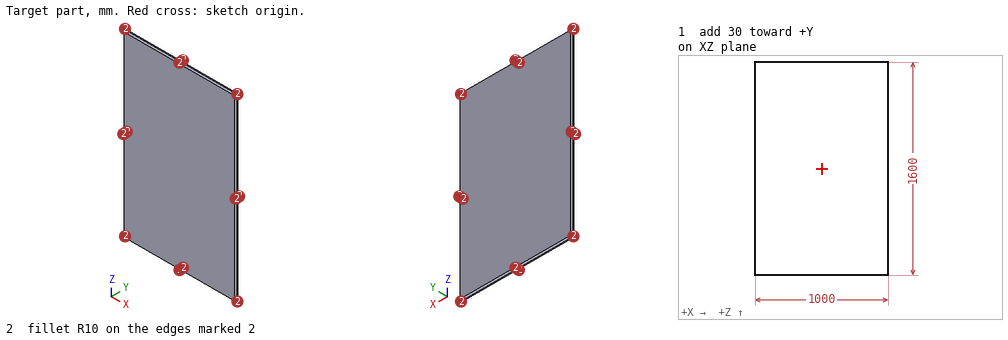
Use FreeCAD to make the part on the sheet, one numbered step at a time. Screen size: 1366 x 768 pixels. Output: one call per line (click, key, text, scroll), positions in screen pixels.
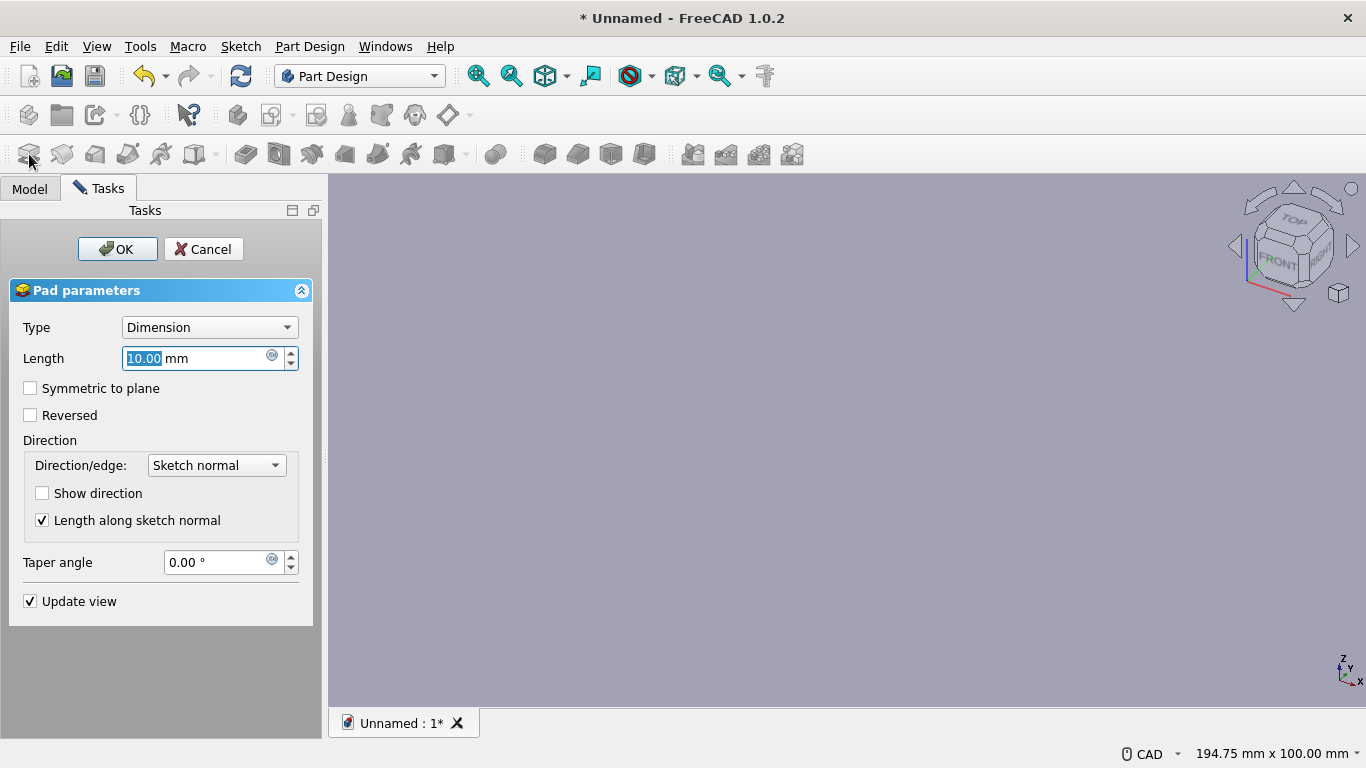
text(30)
key(Tab)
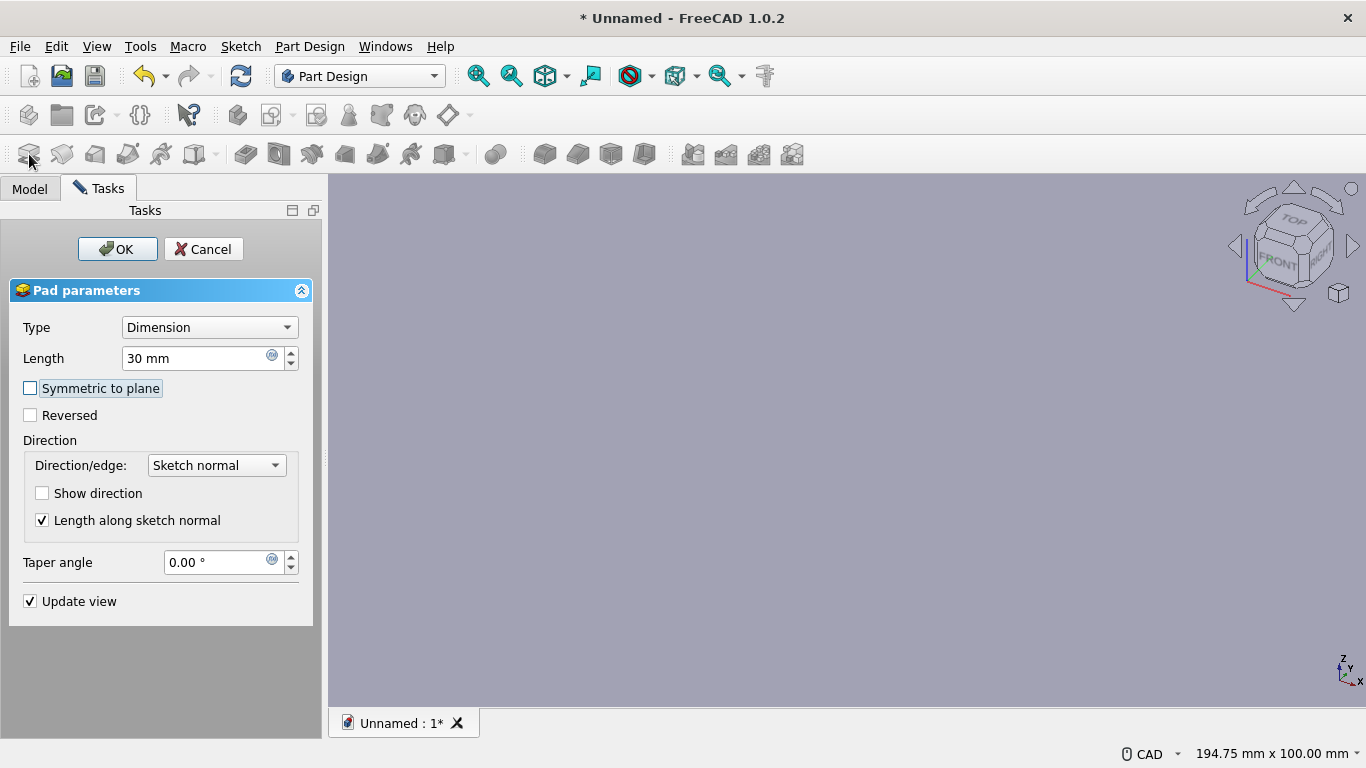
click(31, 415)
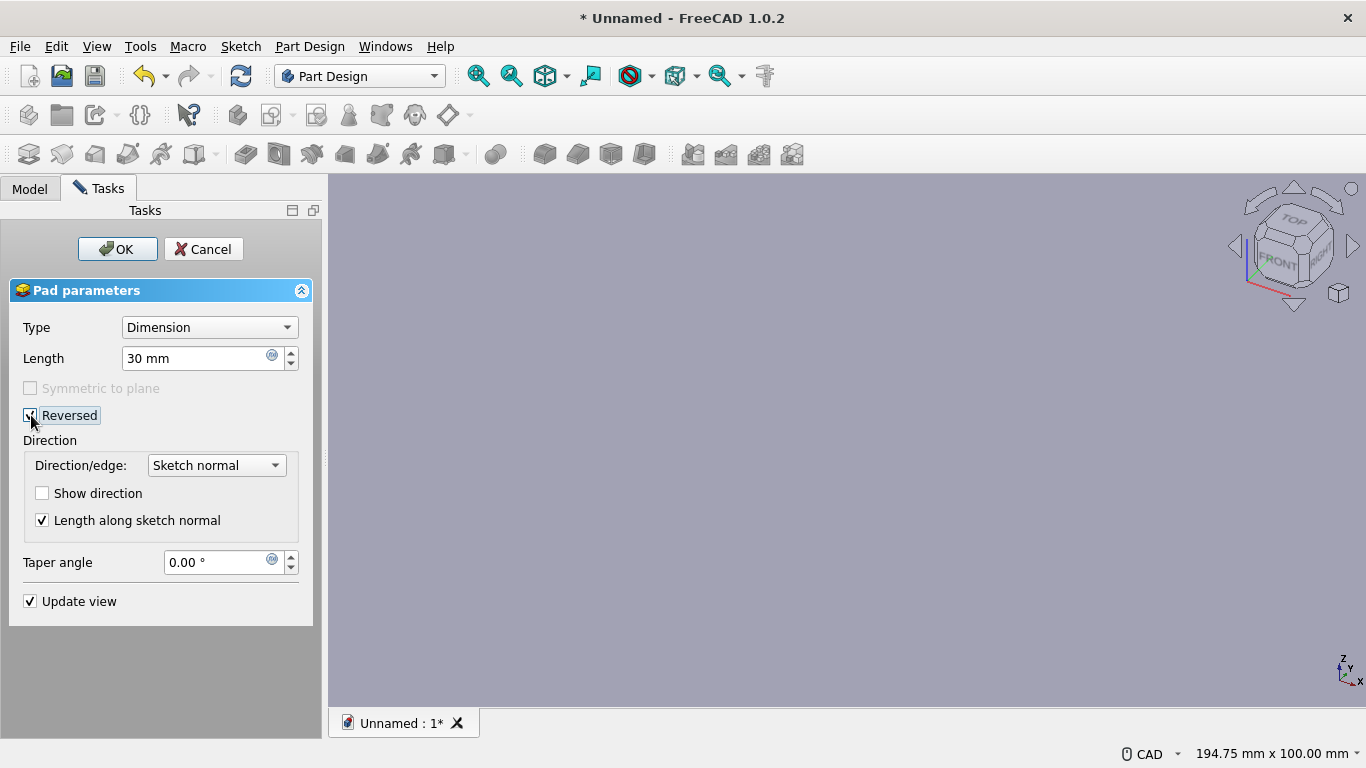
click(118, 249)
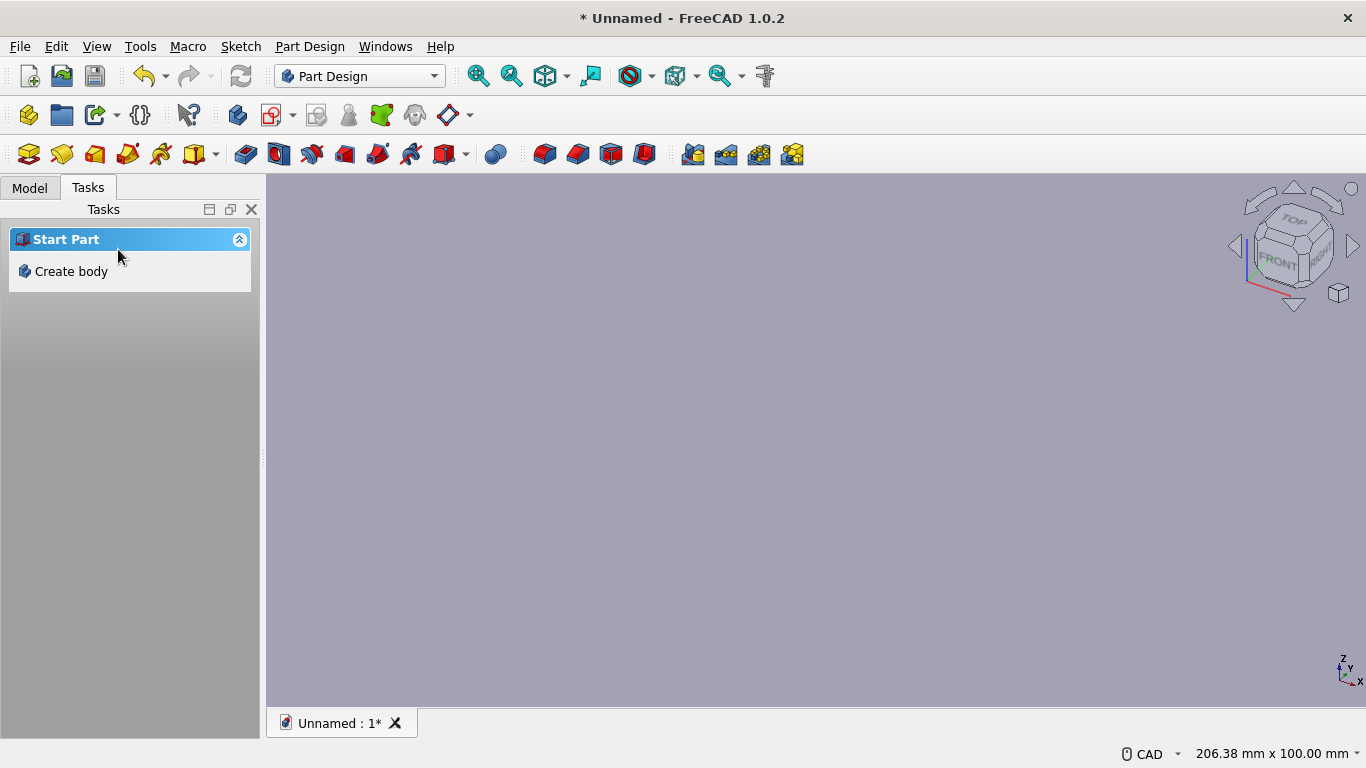
key(v)
key(f)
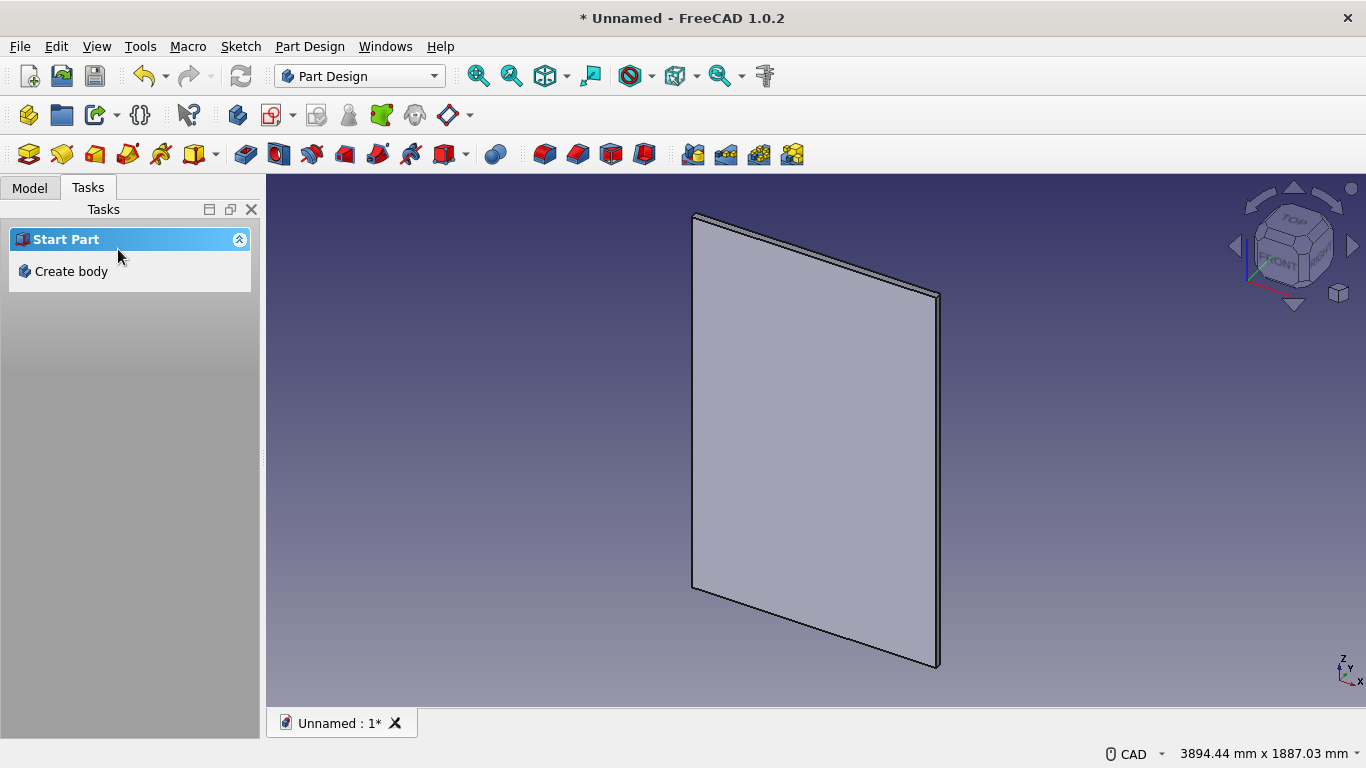
click(814, 389)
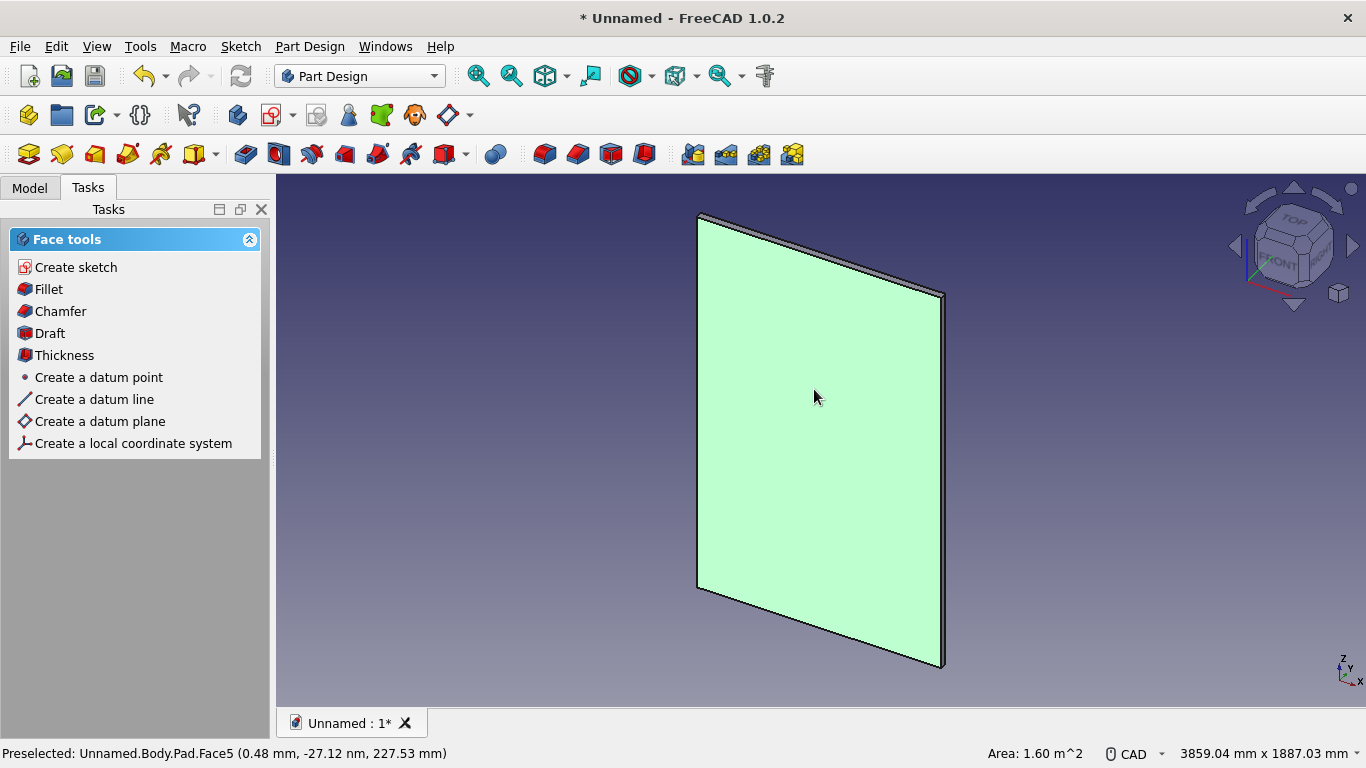
key(0)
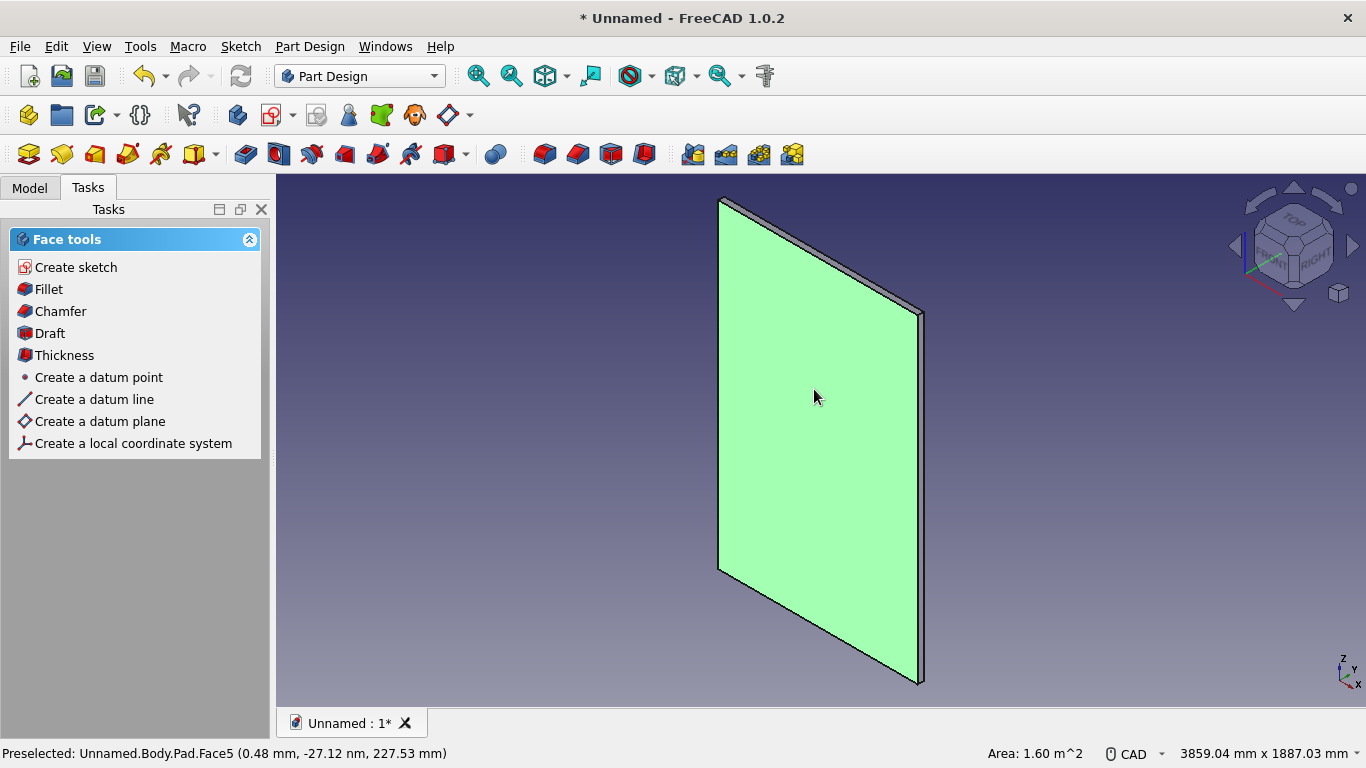
key(2)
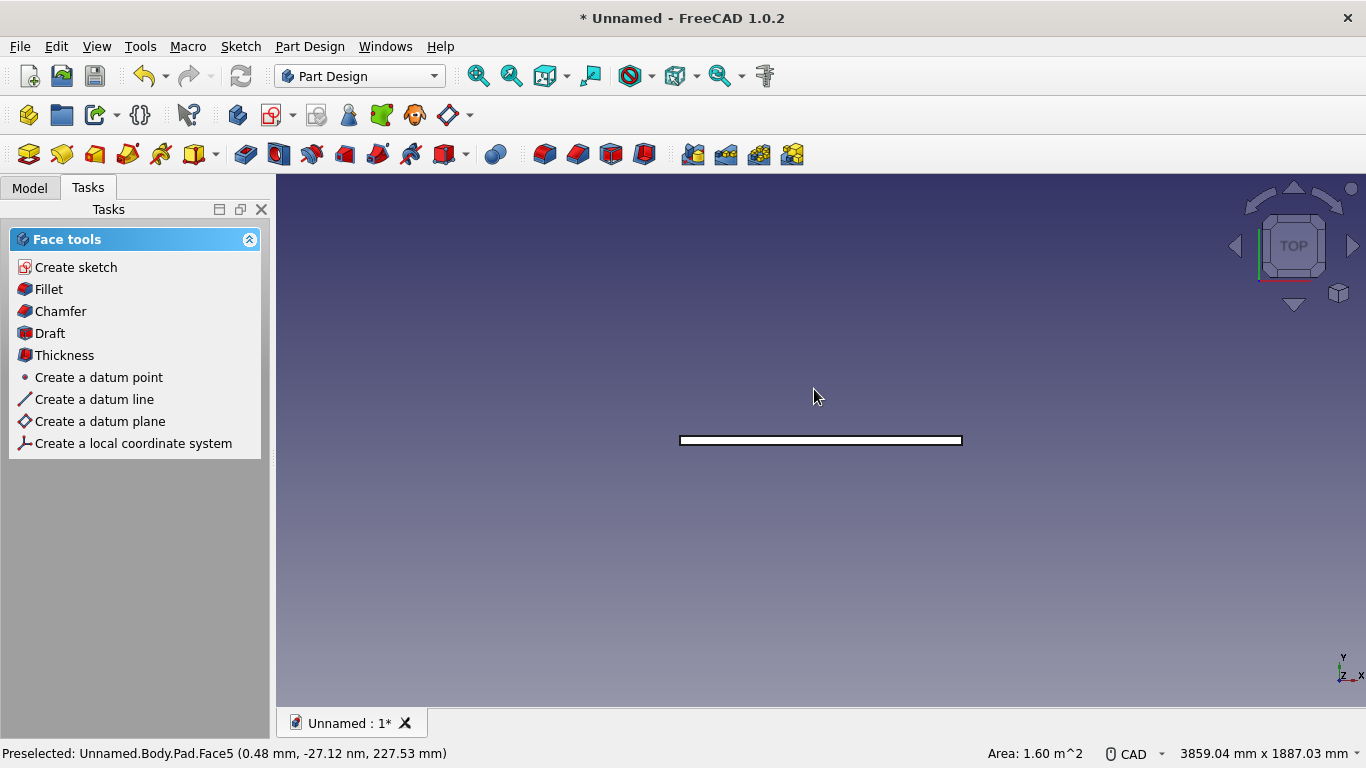
key(v)
key(f)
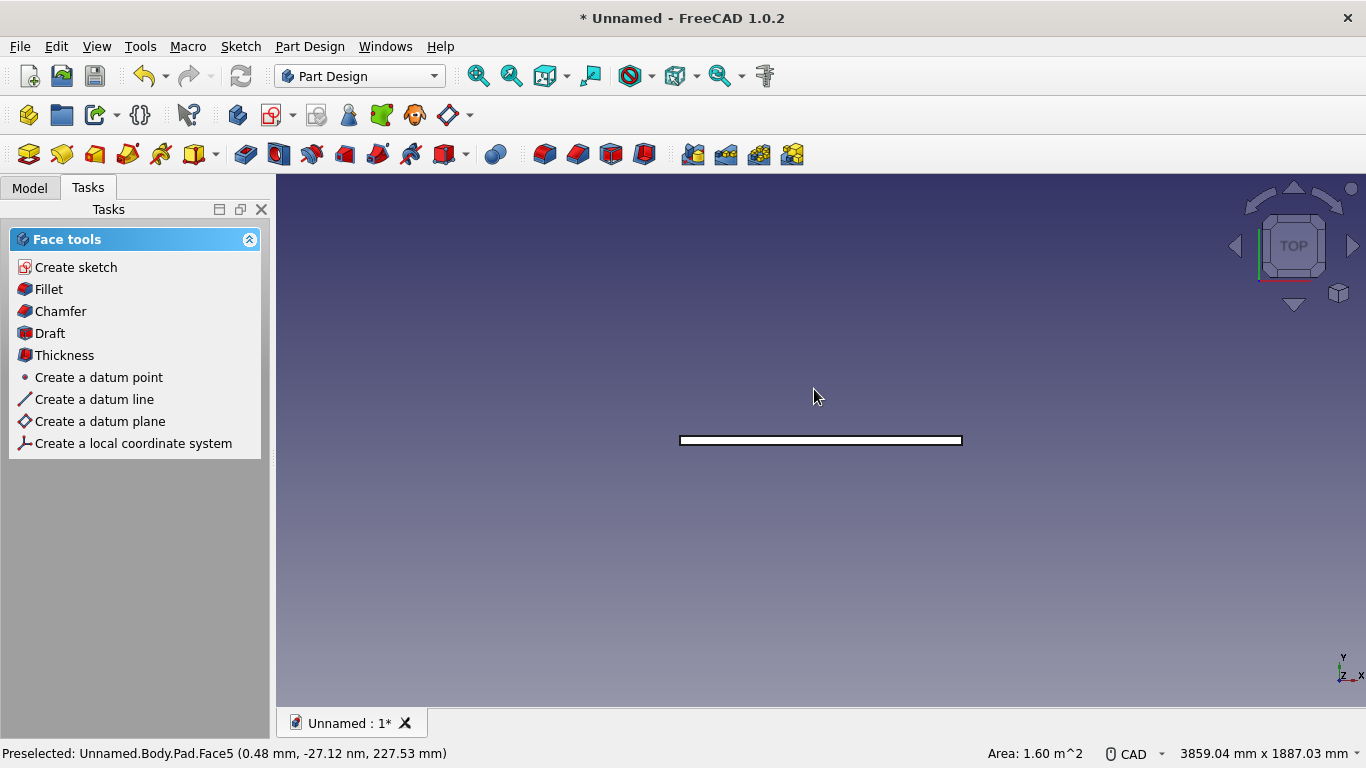
click(962, 442, ctrl)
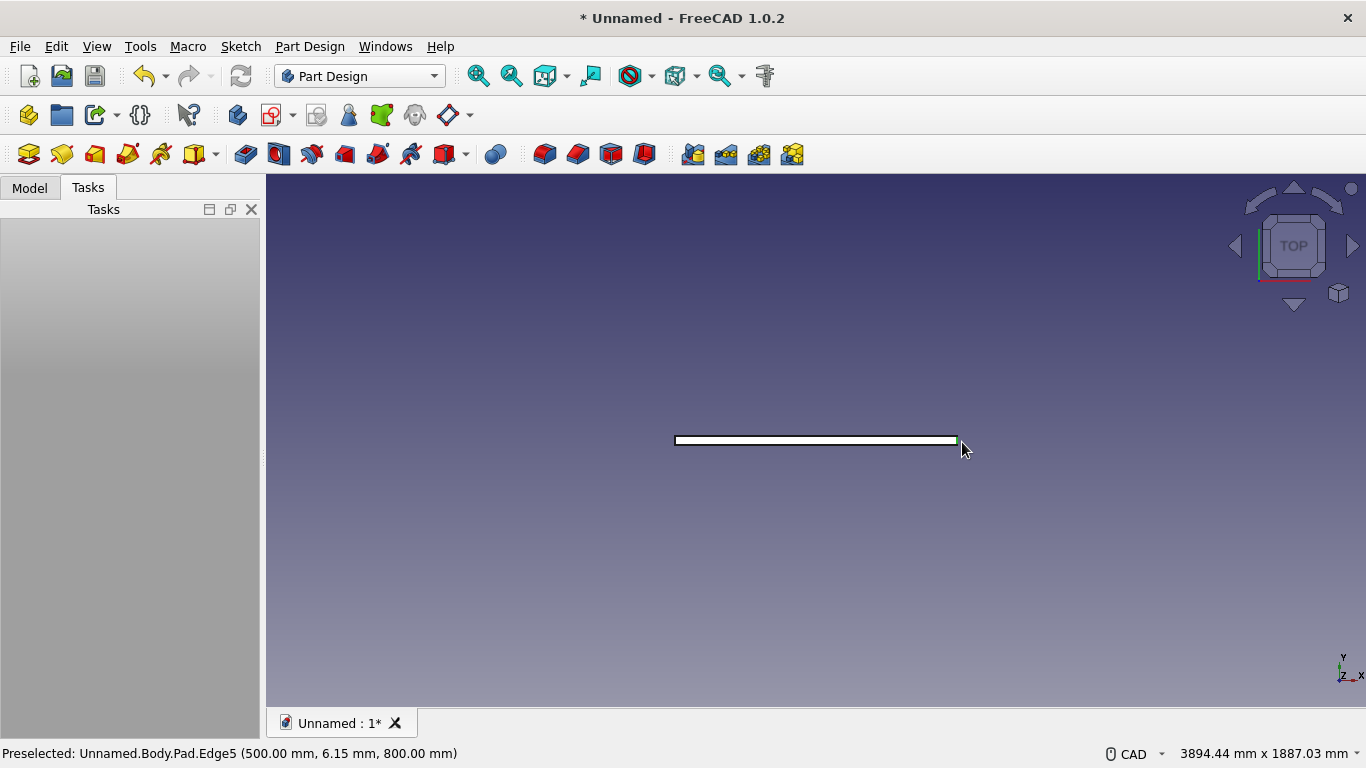
click(675, 442, ctrl)